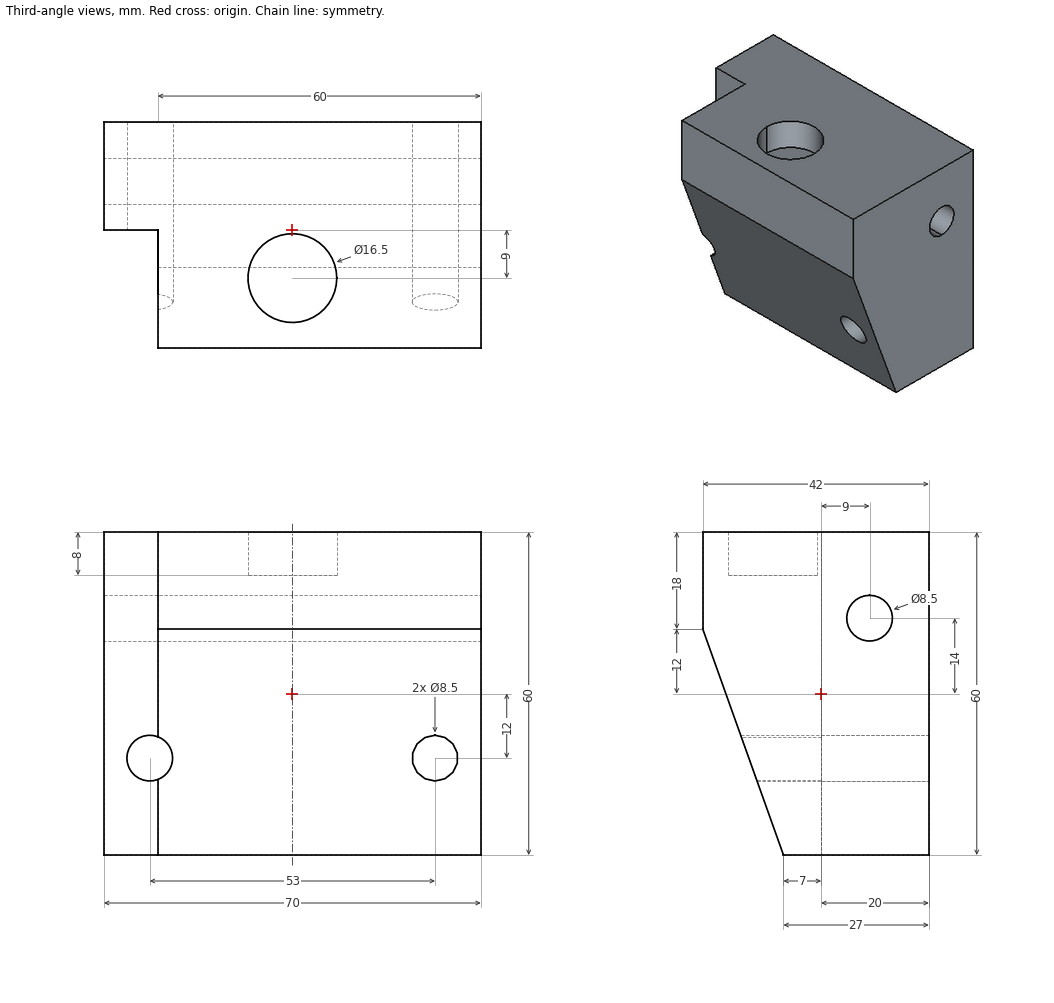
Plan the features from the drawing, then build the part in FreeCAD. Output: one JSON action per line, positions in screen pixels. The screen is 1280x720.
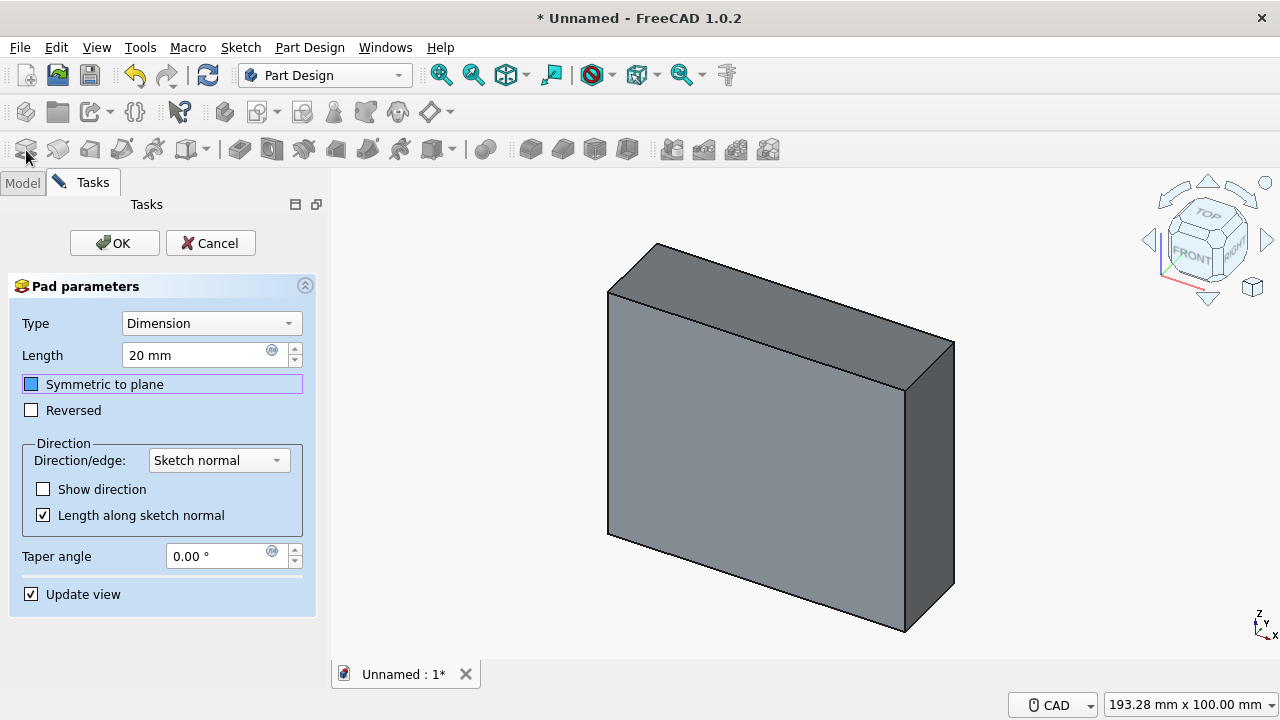
{"action": "left_click", "coordinate": [30, 410]}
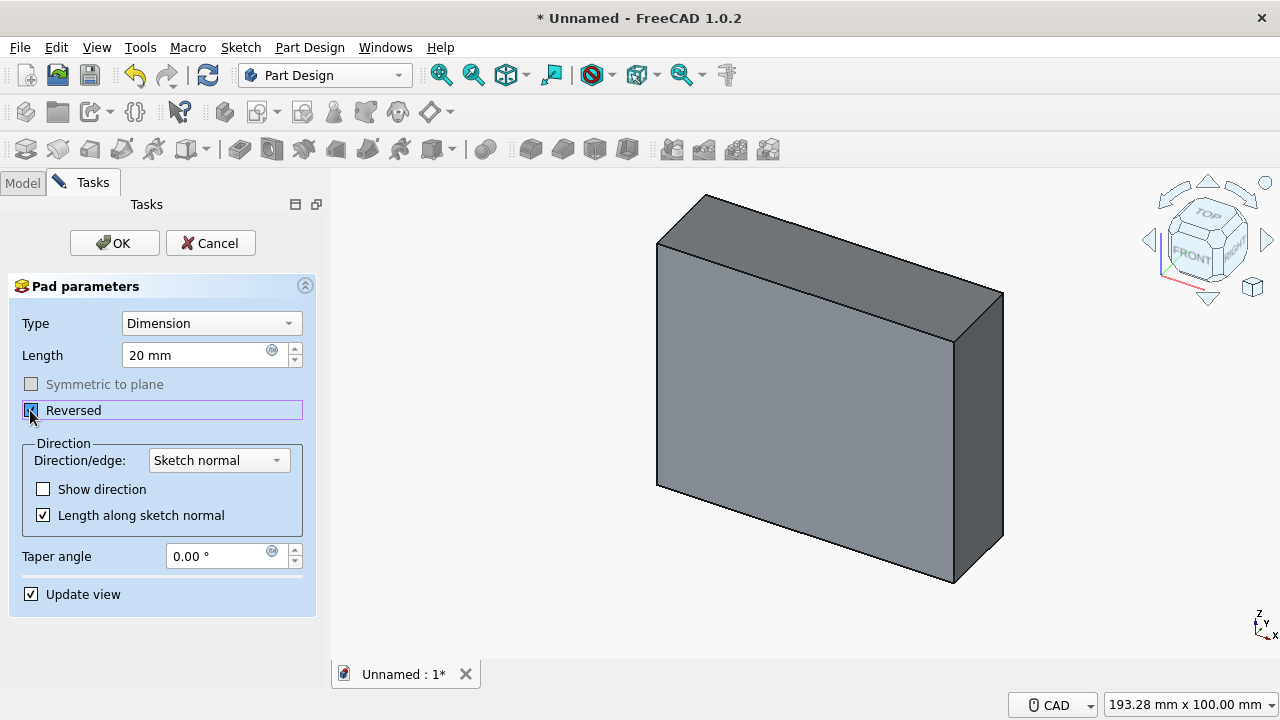
{"action": "left_click", "coordinate": [115, 243]}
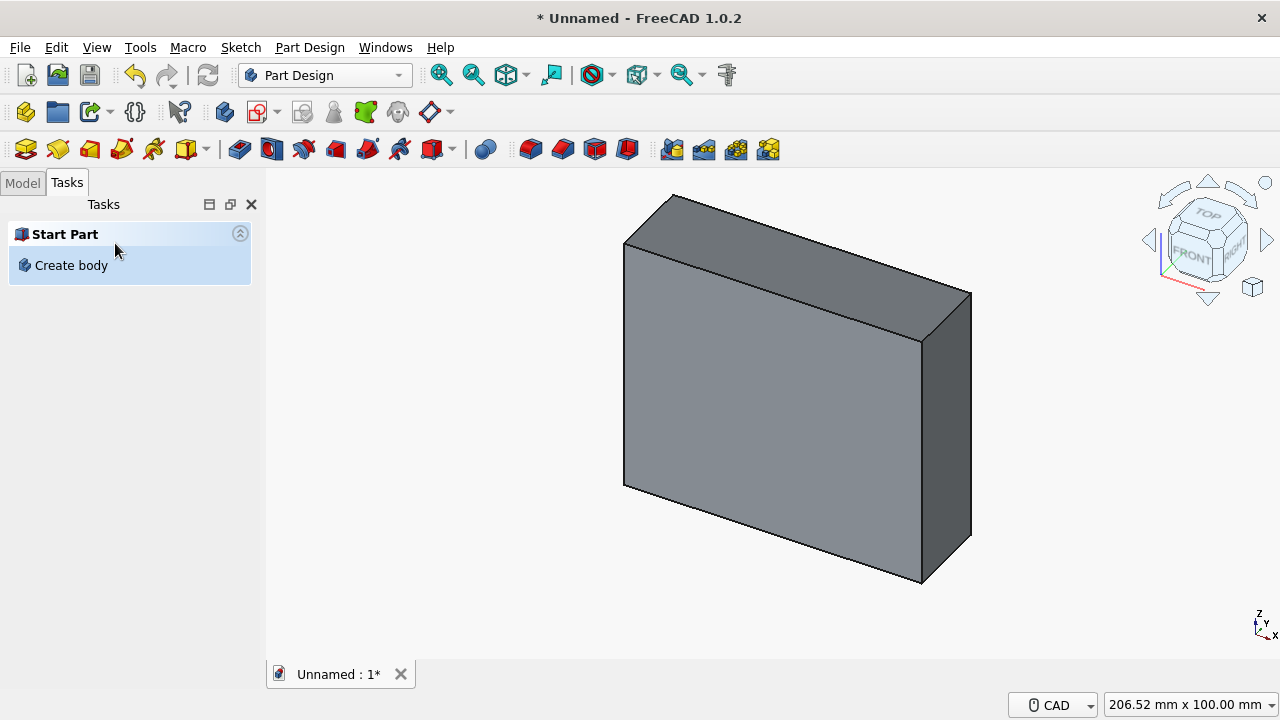
{"action": "left_click", "coordinate": [946, 368]}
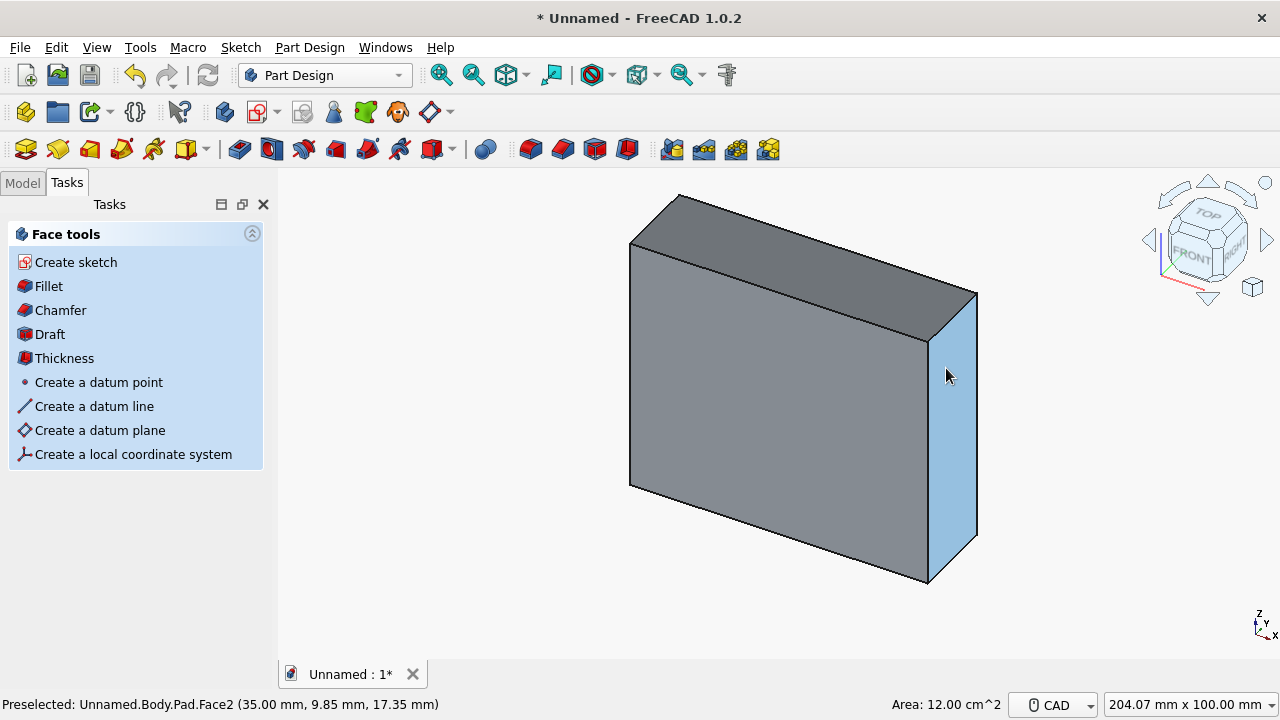
{"action": "left_click", "coordinate": [258, 112]}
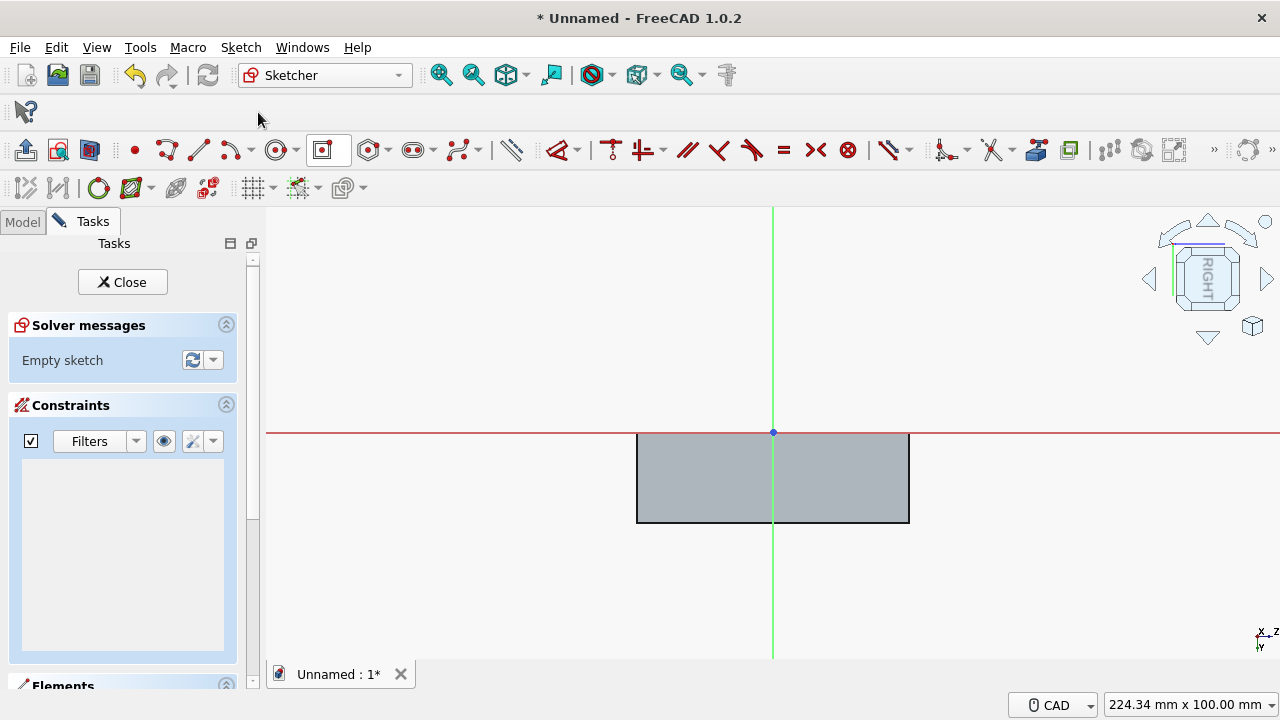
{"action": "scroll", "coordinate": [912, 419], "scroll_direction": "up", "scroll_amount": 2}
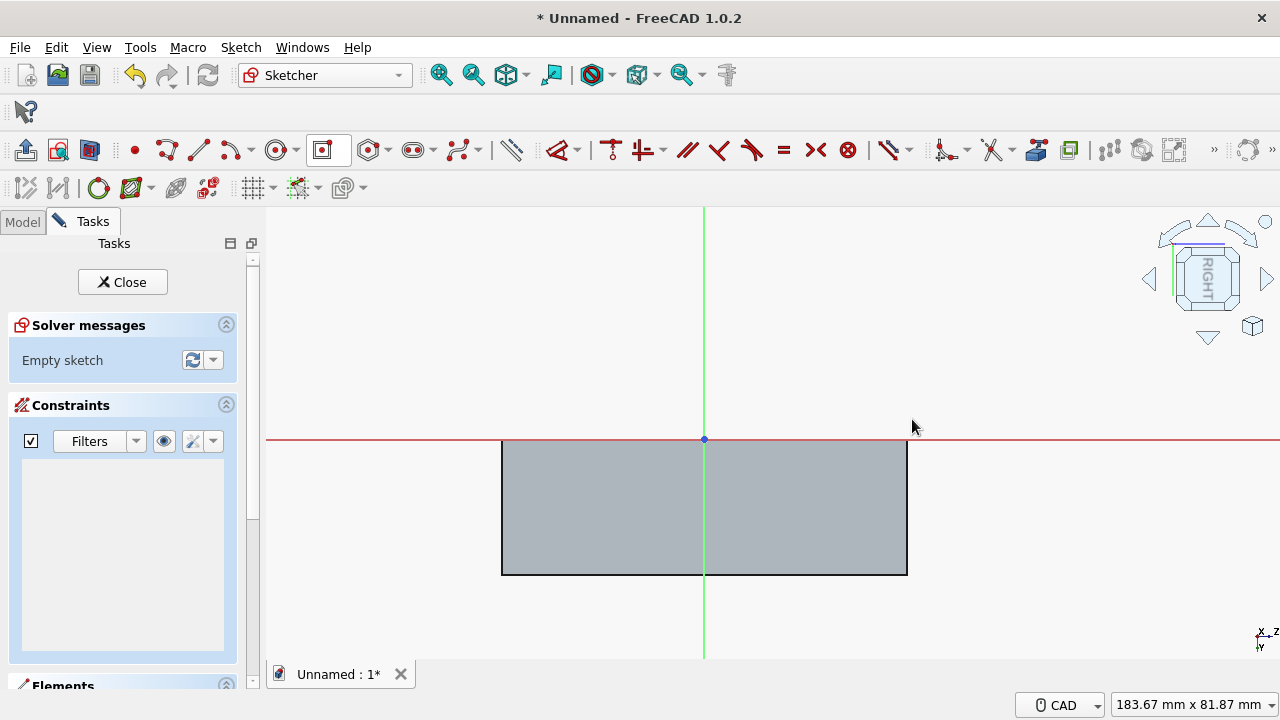
{"action": "key", "text": "g m"}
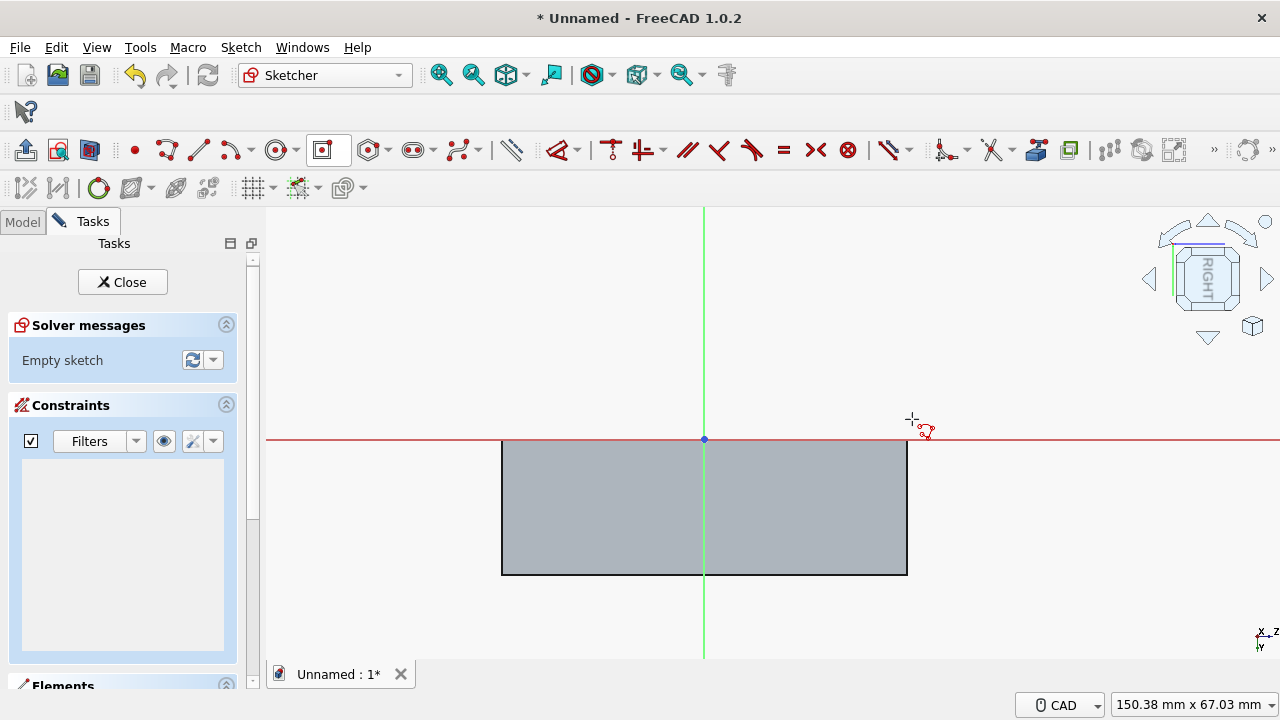
{"action": "left_click", "coordinate": [785, 291]}
{"action": "left_click", "coordinate": [502, 392]}
{"action": "left_click", "coordinate": [502, 575]}
{"action": "left_click", "coordinate": [907, 575]}
{"action": "left_click", "coordinate": [907, 291]}
{"action": "left_click", "coordinate": [785, 292]}
{"action": "key", "text": "Escape"}
{"action": "key", "text": "Escape"}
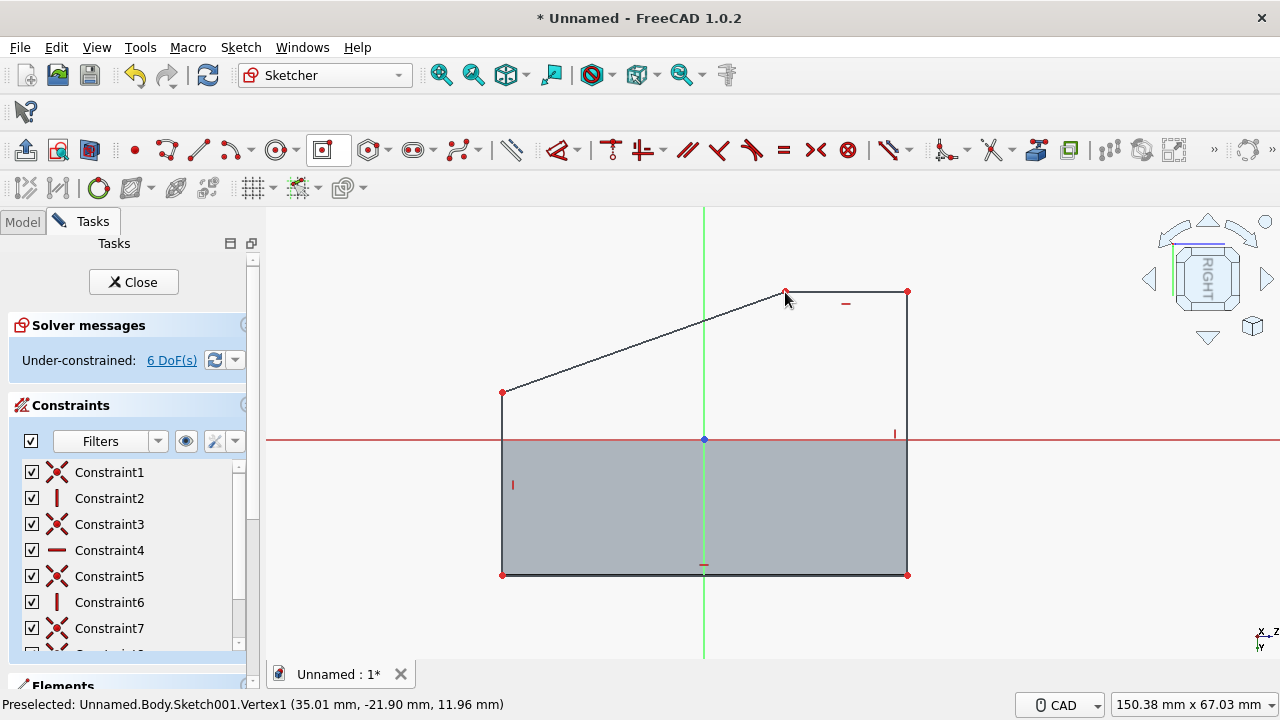
{"action": "left_click", "coordinate": [502, 521]}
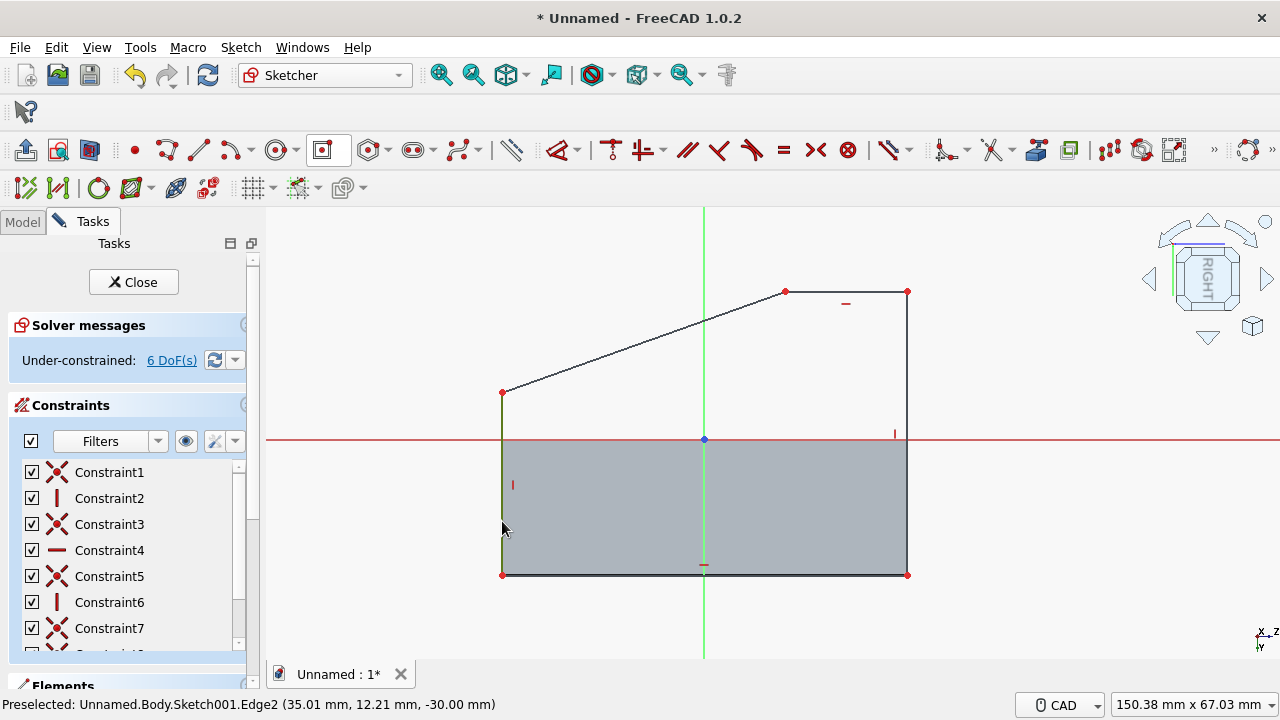
{"action": "key", "text": "i"}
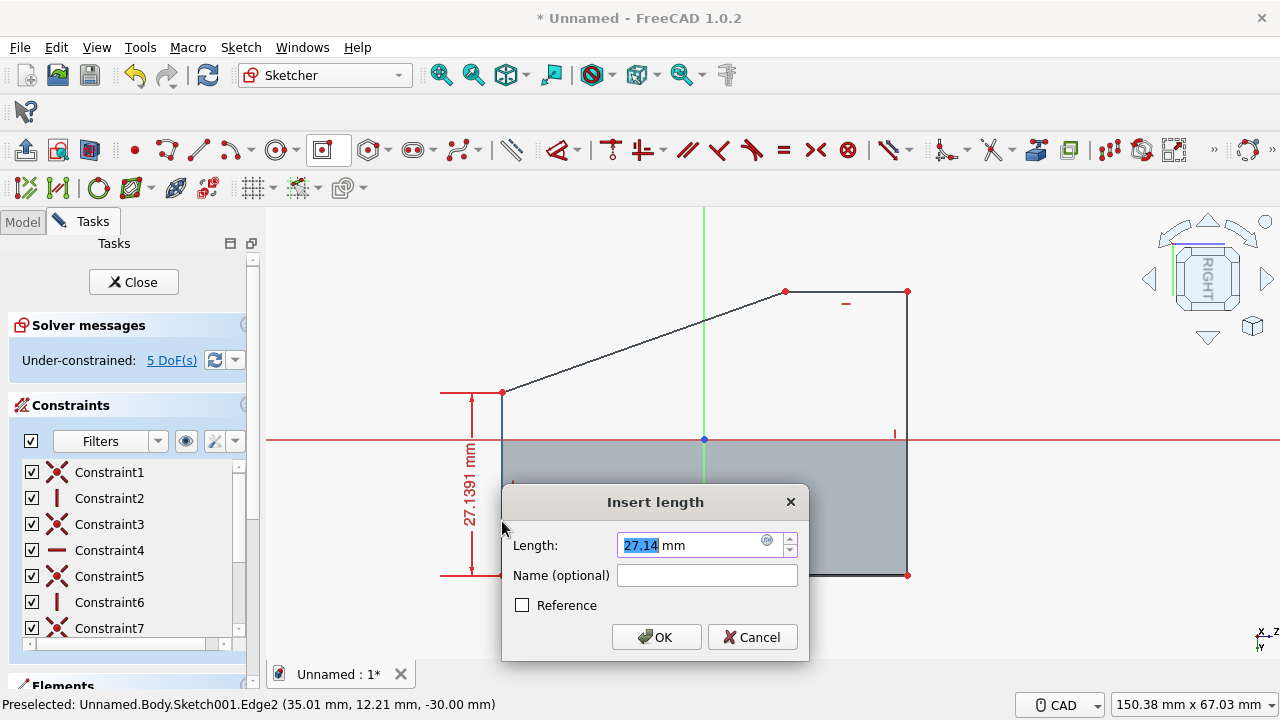
{"action": "type", "text": "27"}
{"action": "key", "text": "Return"}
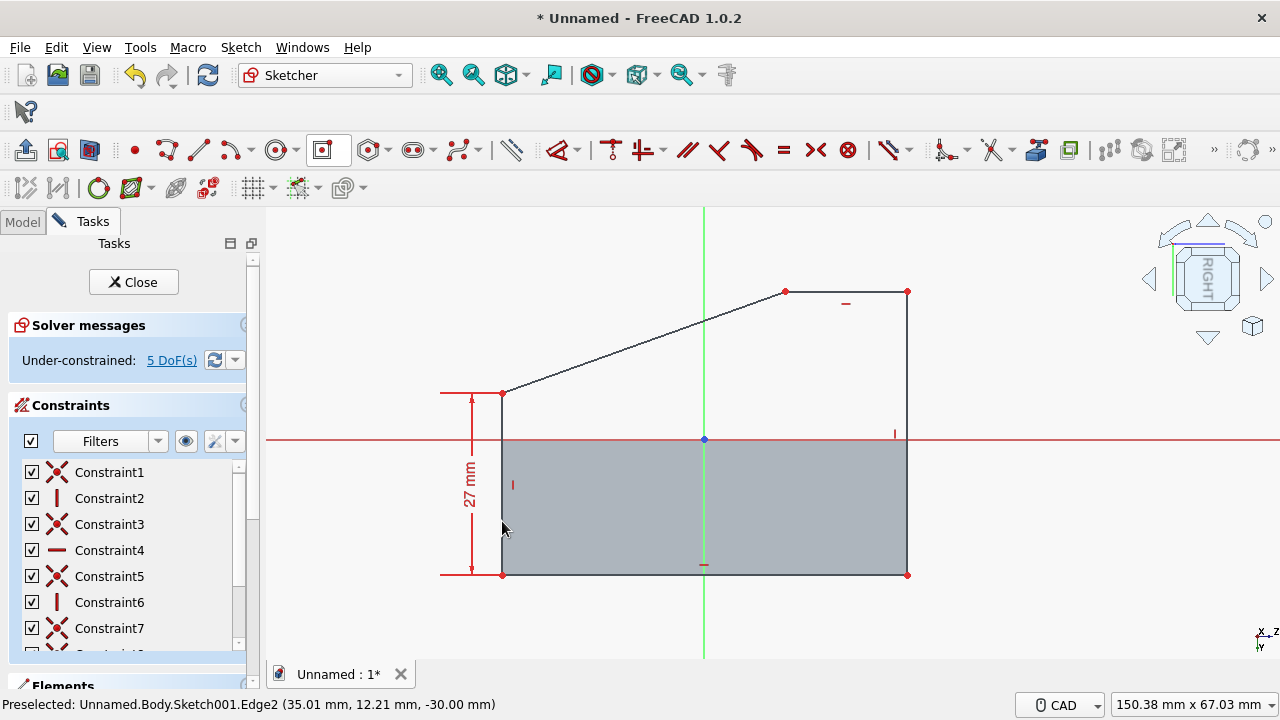
{"action": "left_click", "coordinate": [623, 575]}